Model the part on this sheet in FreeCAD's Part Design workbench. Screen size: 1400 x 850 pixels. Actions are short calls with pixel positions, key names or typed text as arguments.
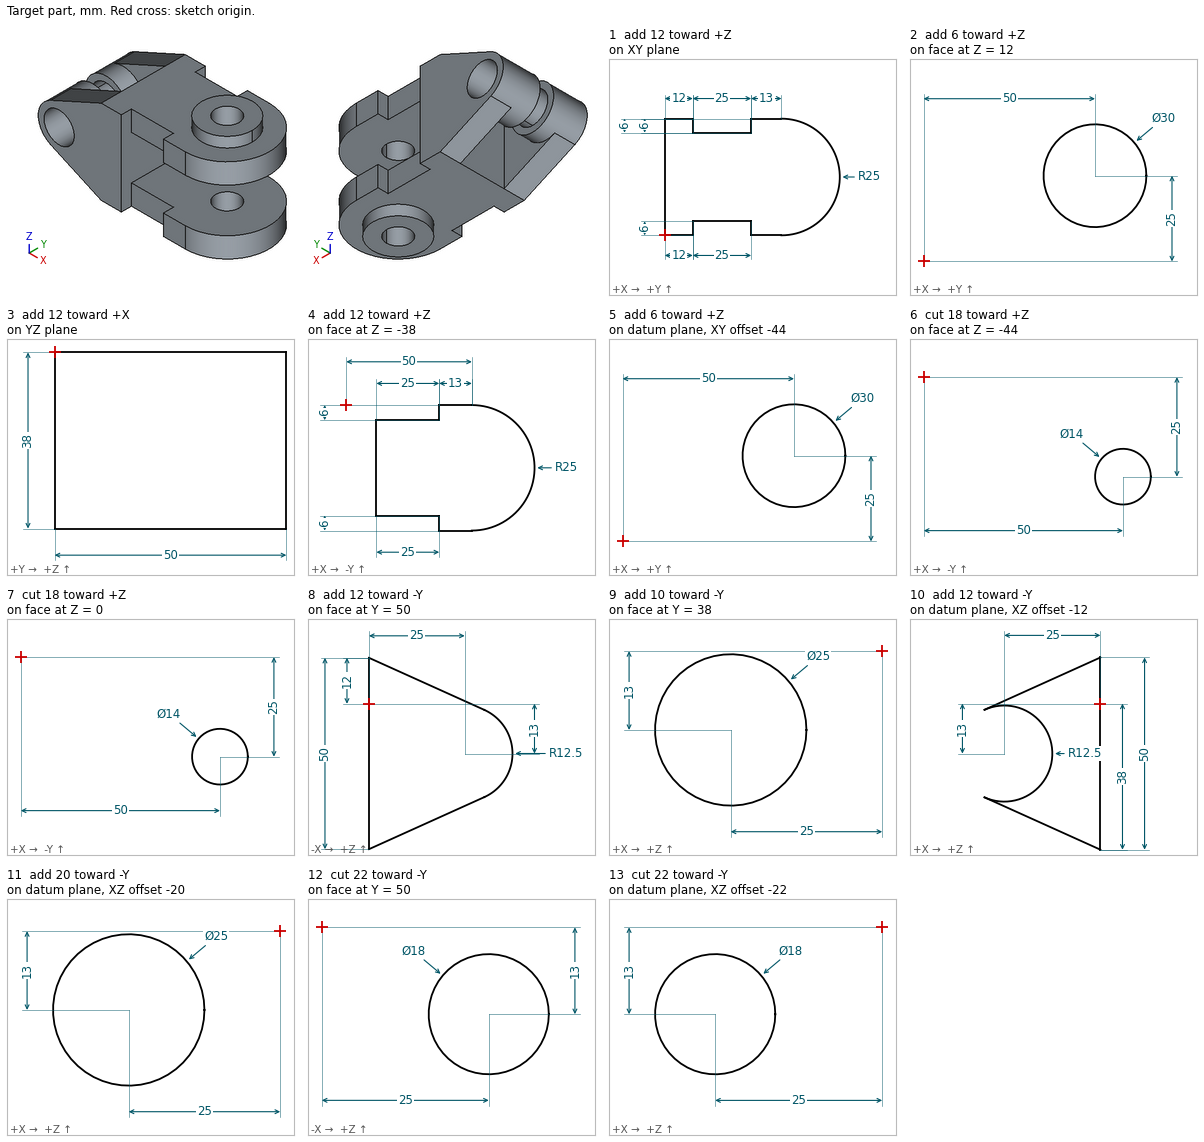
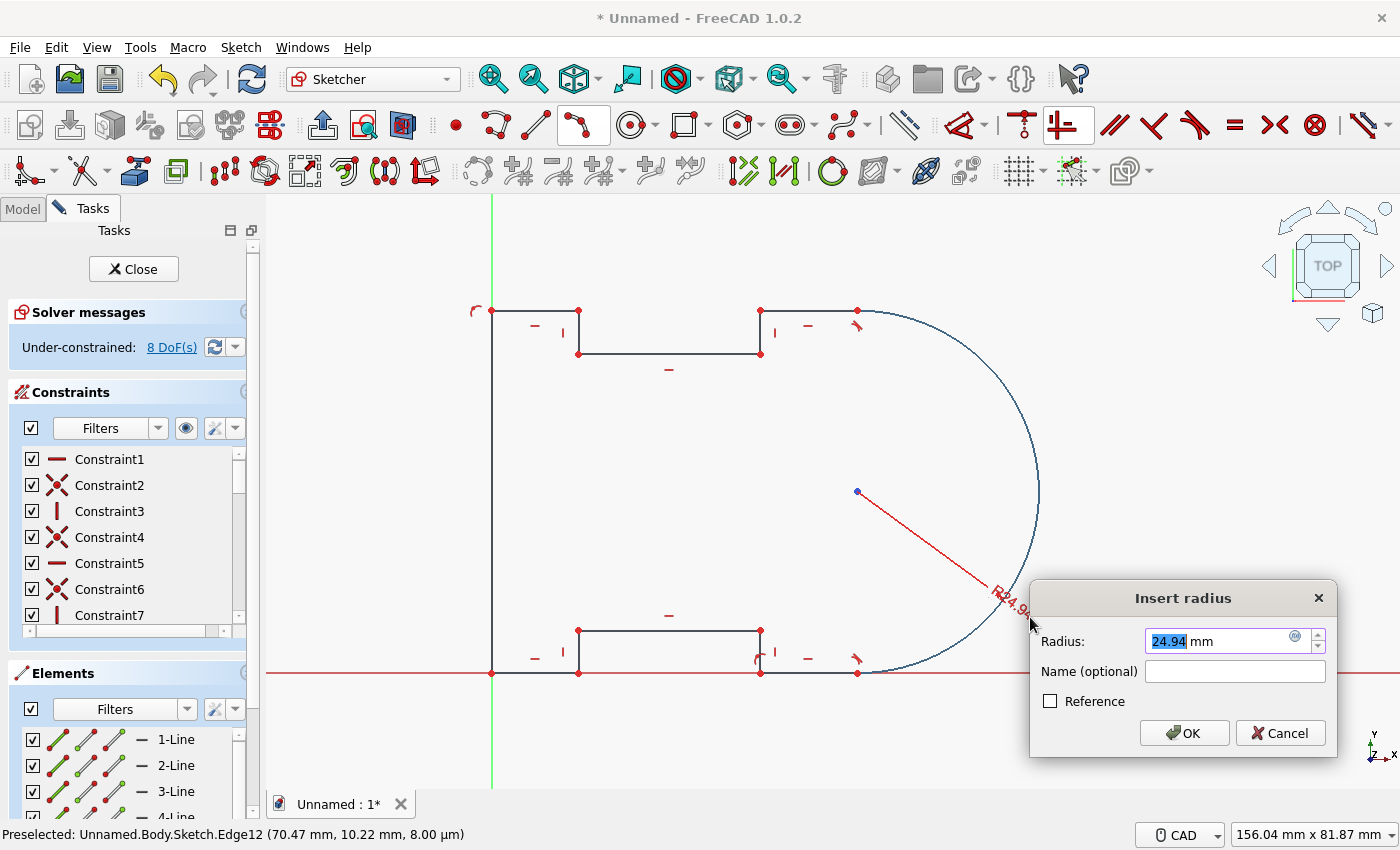
text(25)
key(Return)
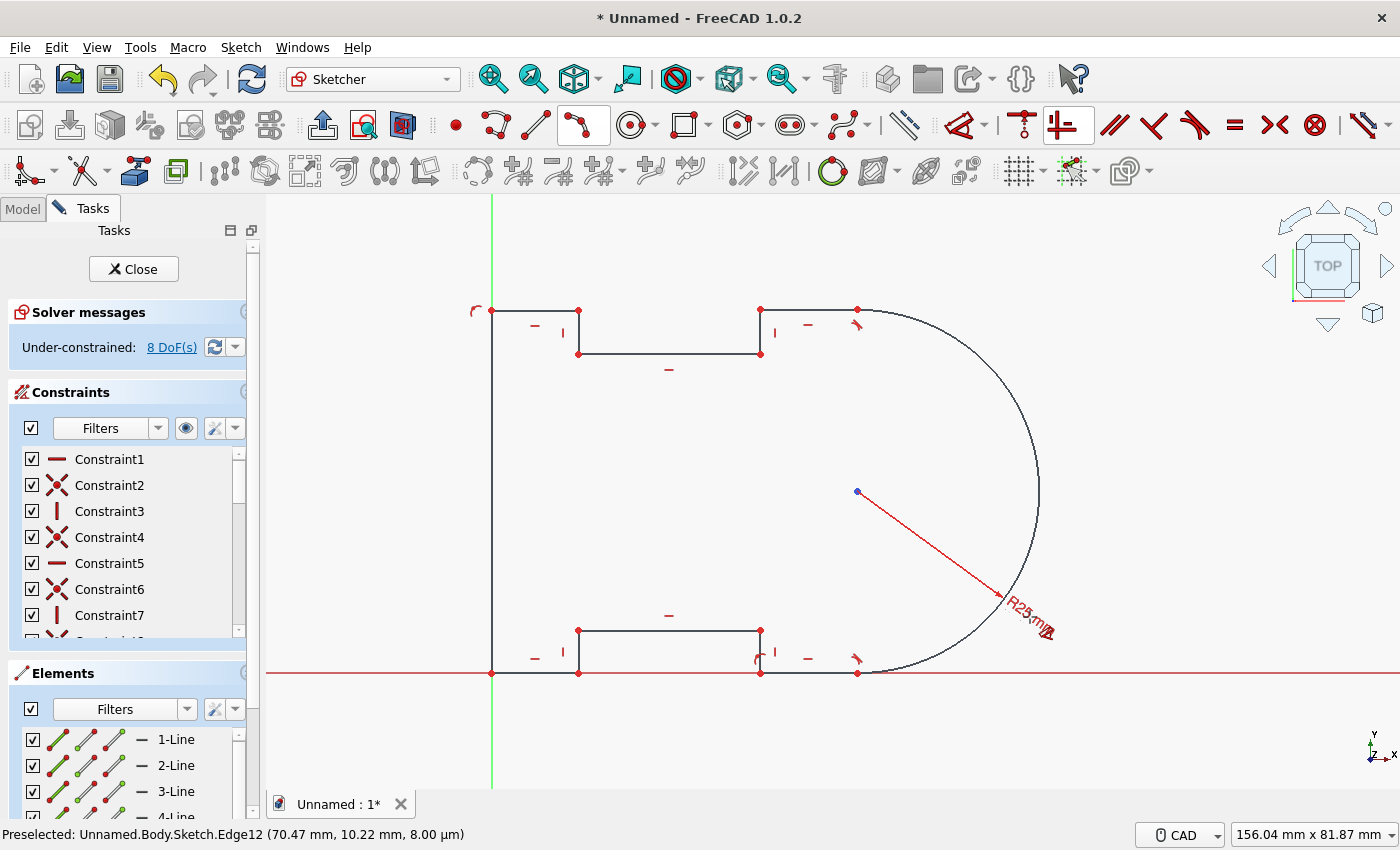
click(760, 323)
click(726, 332)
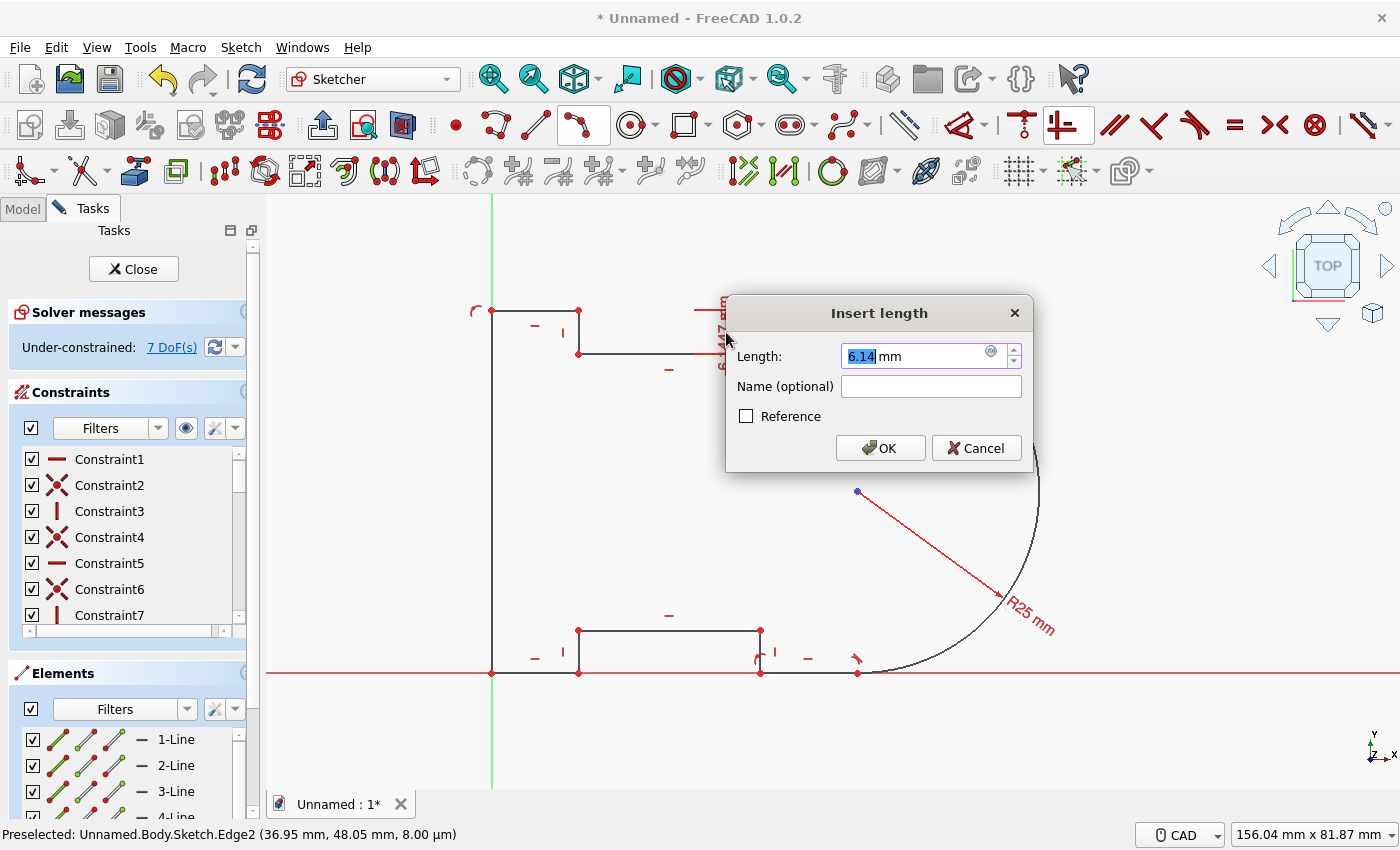
text(6)
key(Return)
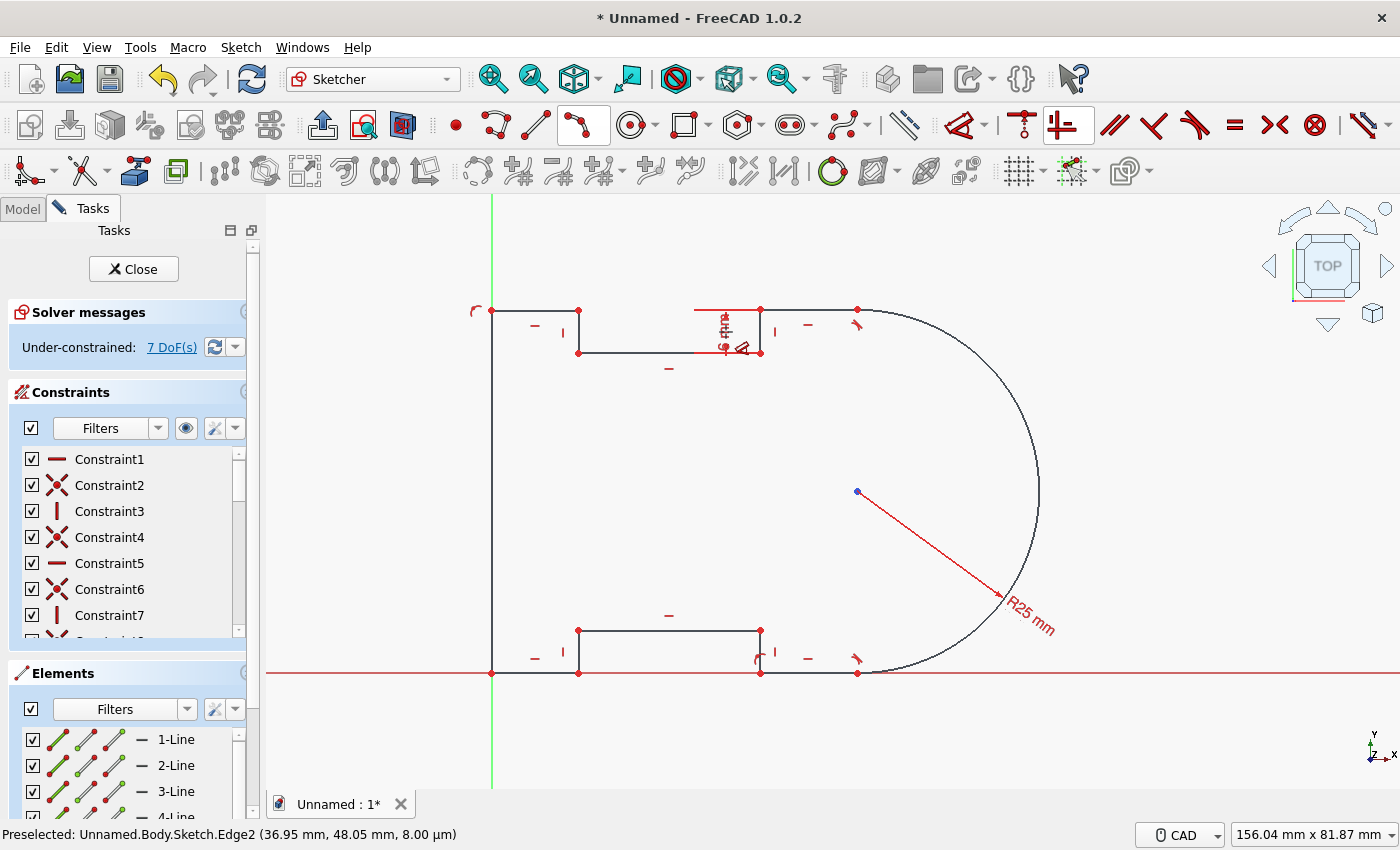
click(579, 341)
click(545, 332)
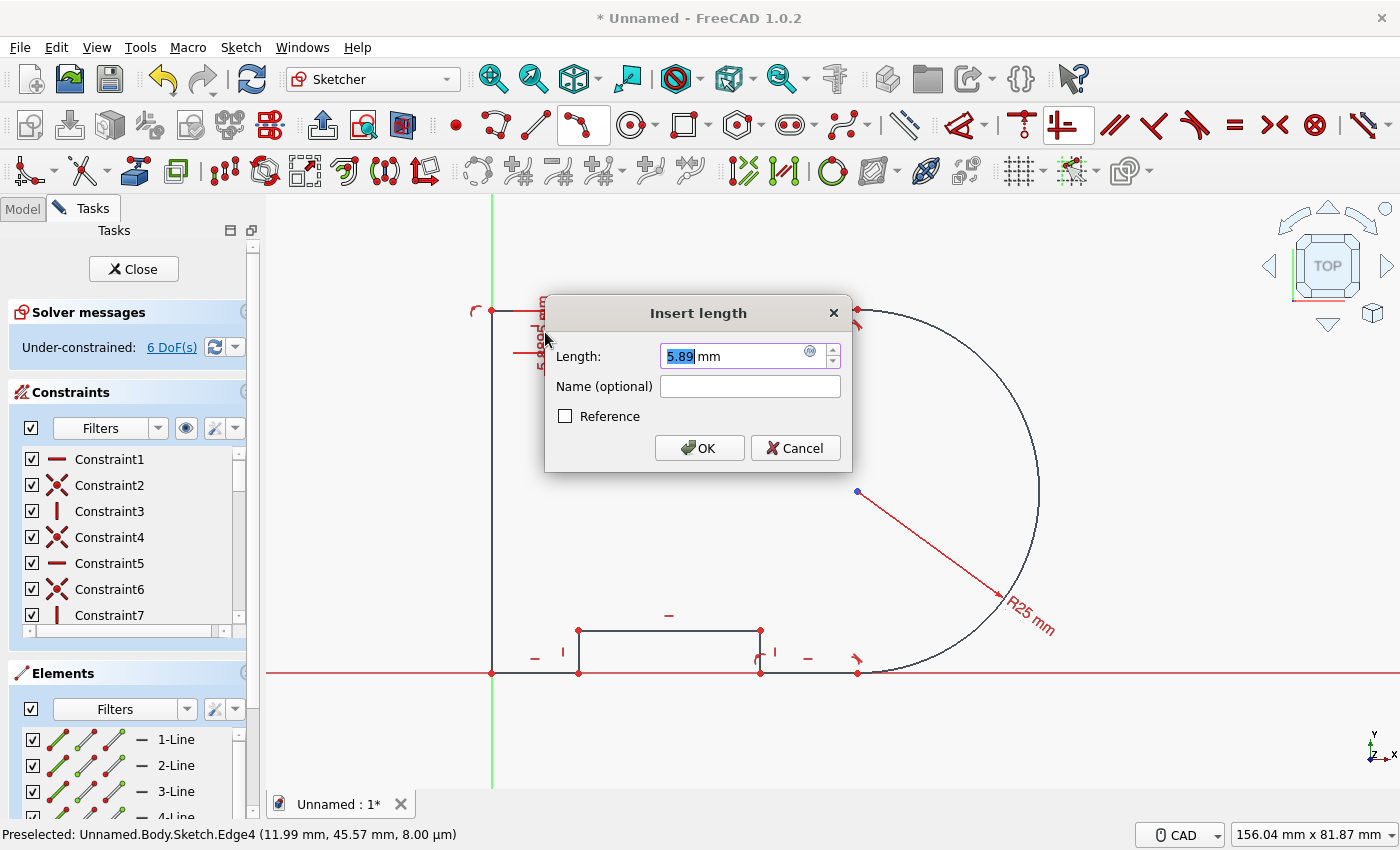
text(6)
key(Return)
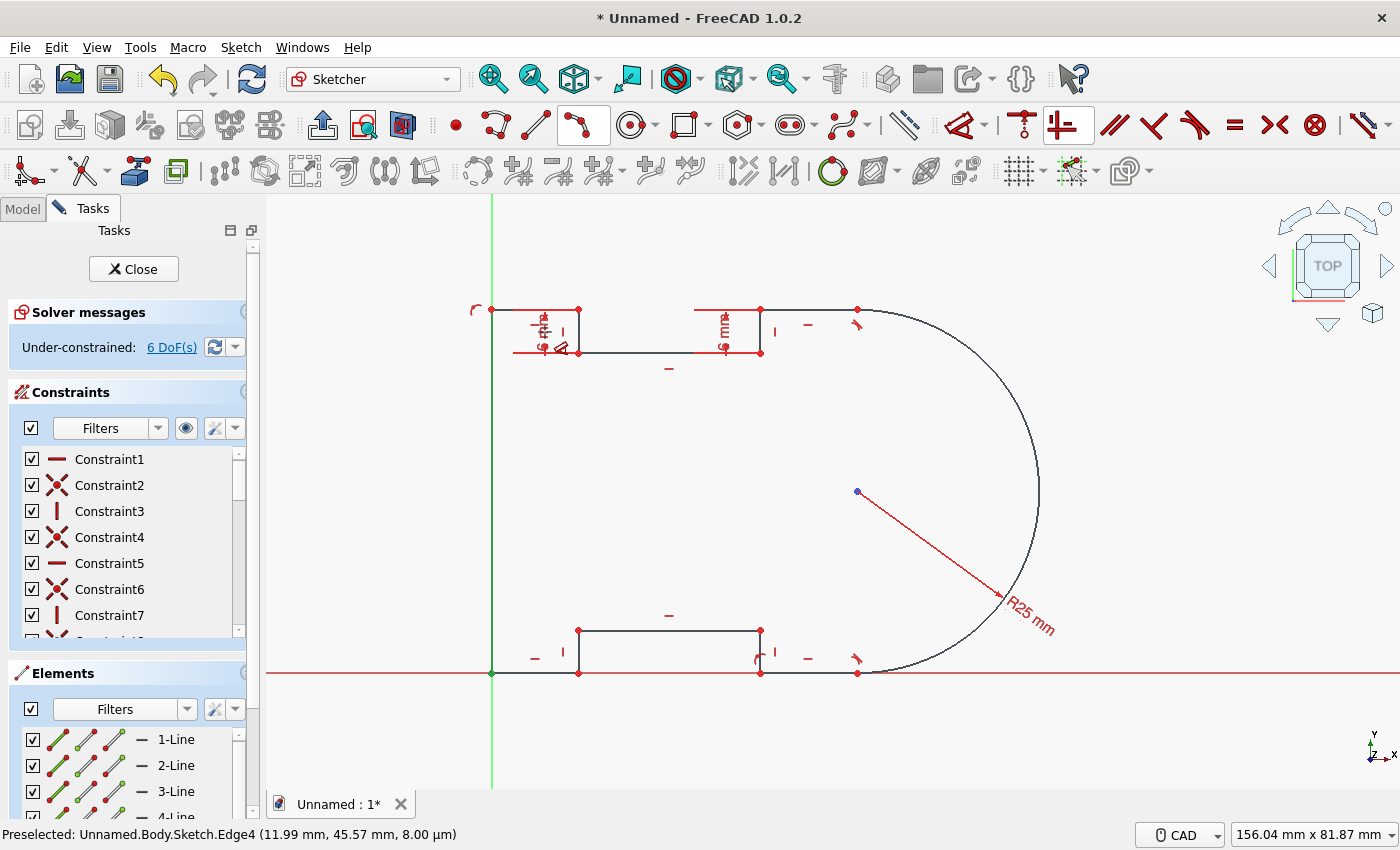
click(579, 660)
click(545, 652)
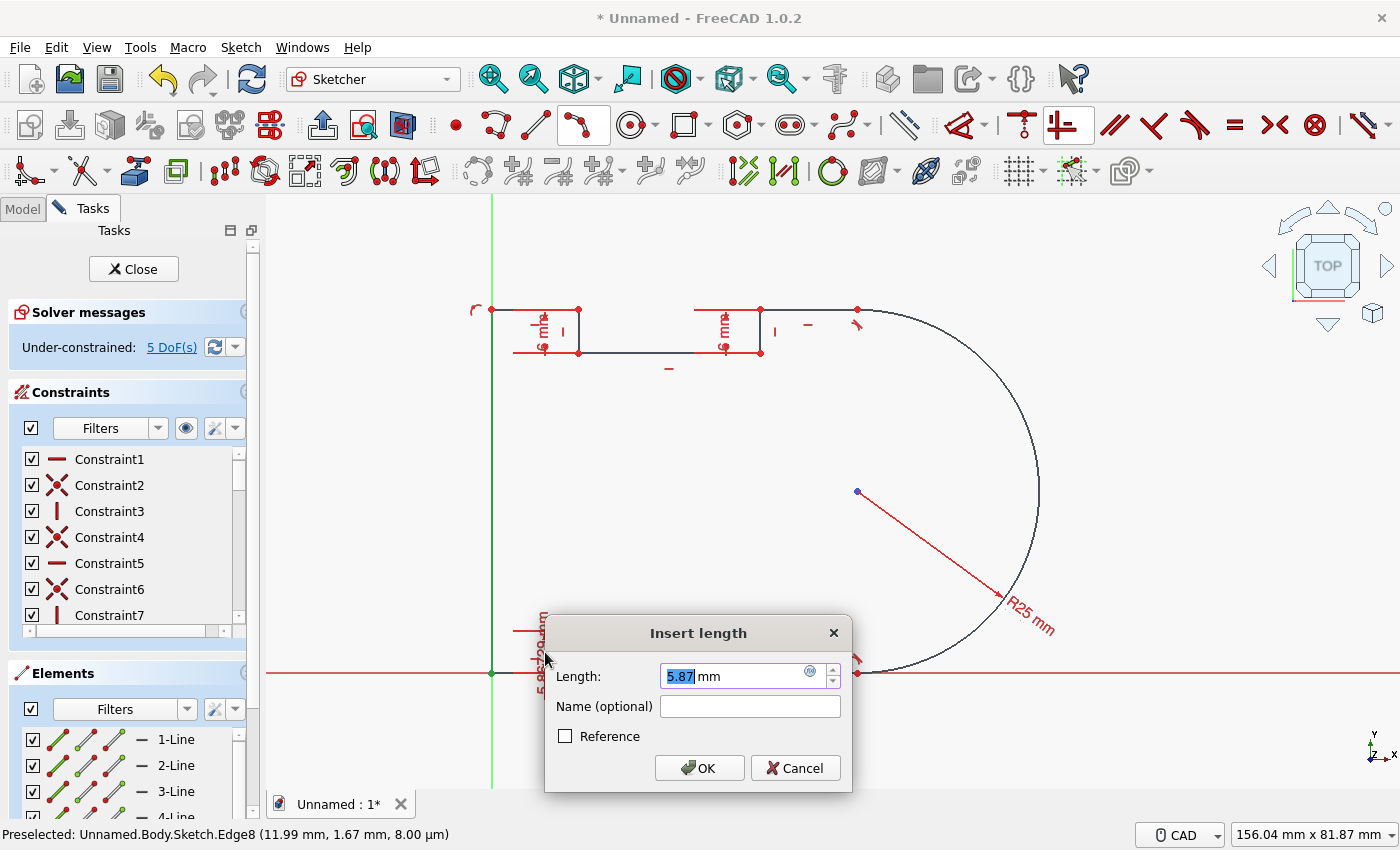
text(6)
key(Return)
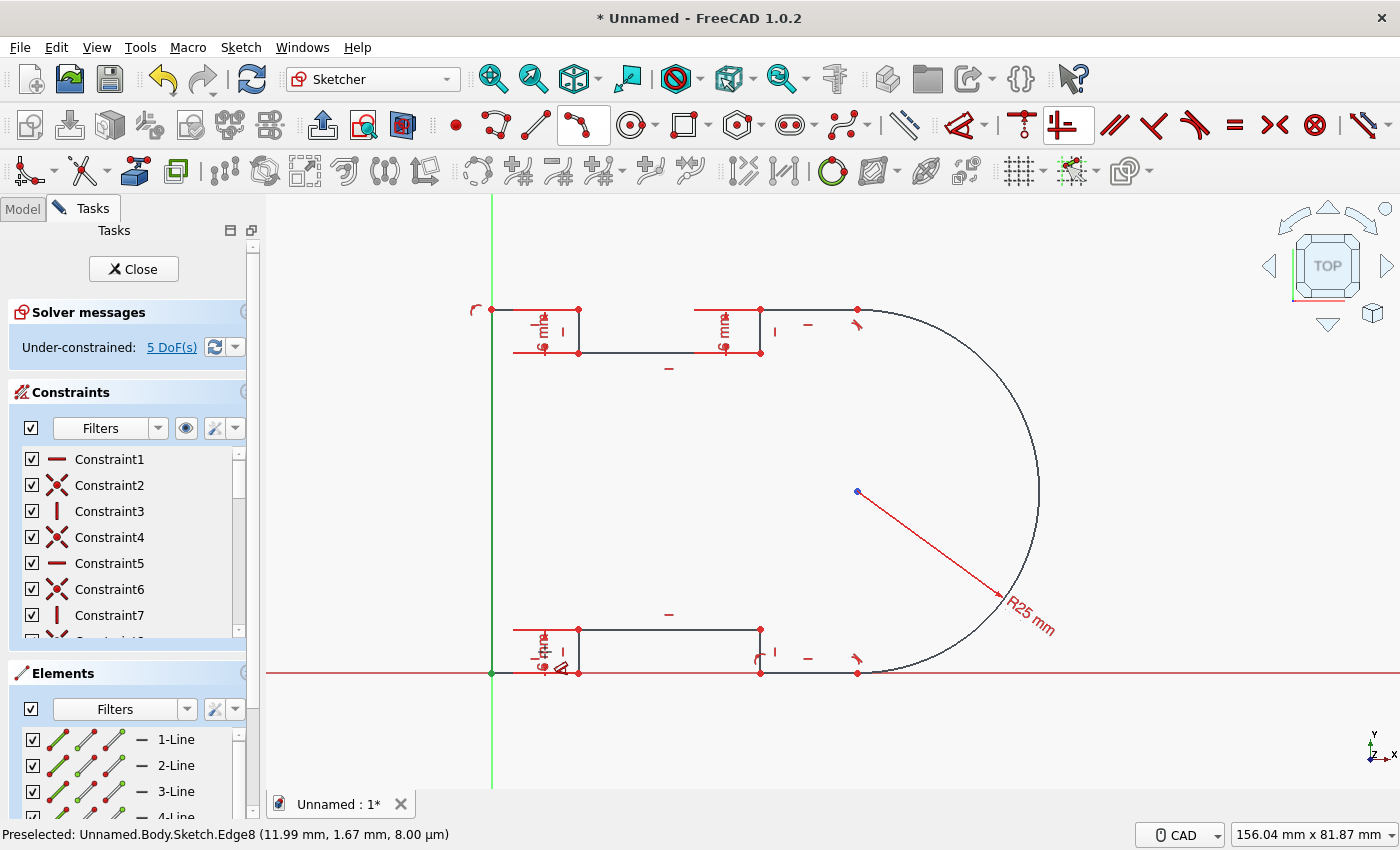
click(828, 310)
click(809, 276)